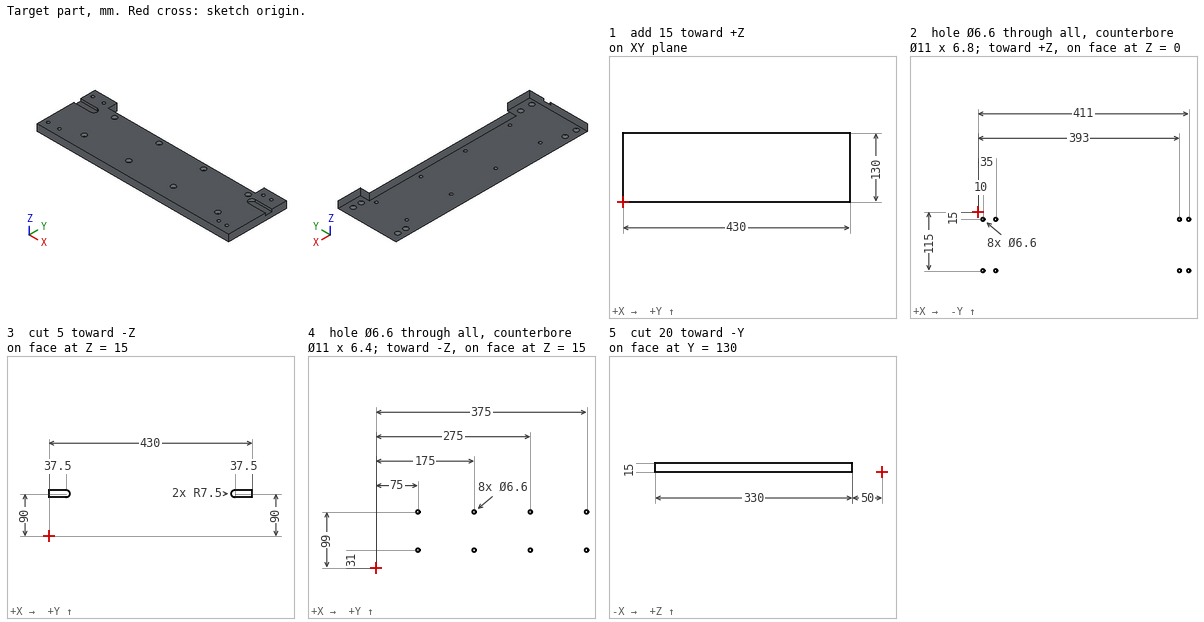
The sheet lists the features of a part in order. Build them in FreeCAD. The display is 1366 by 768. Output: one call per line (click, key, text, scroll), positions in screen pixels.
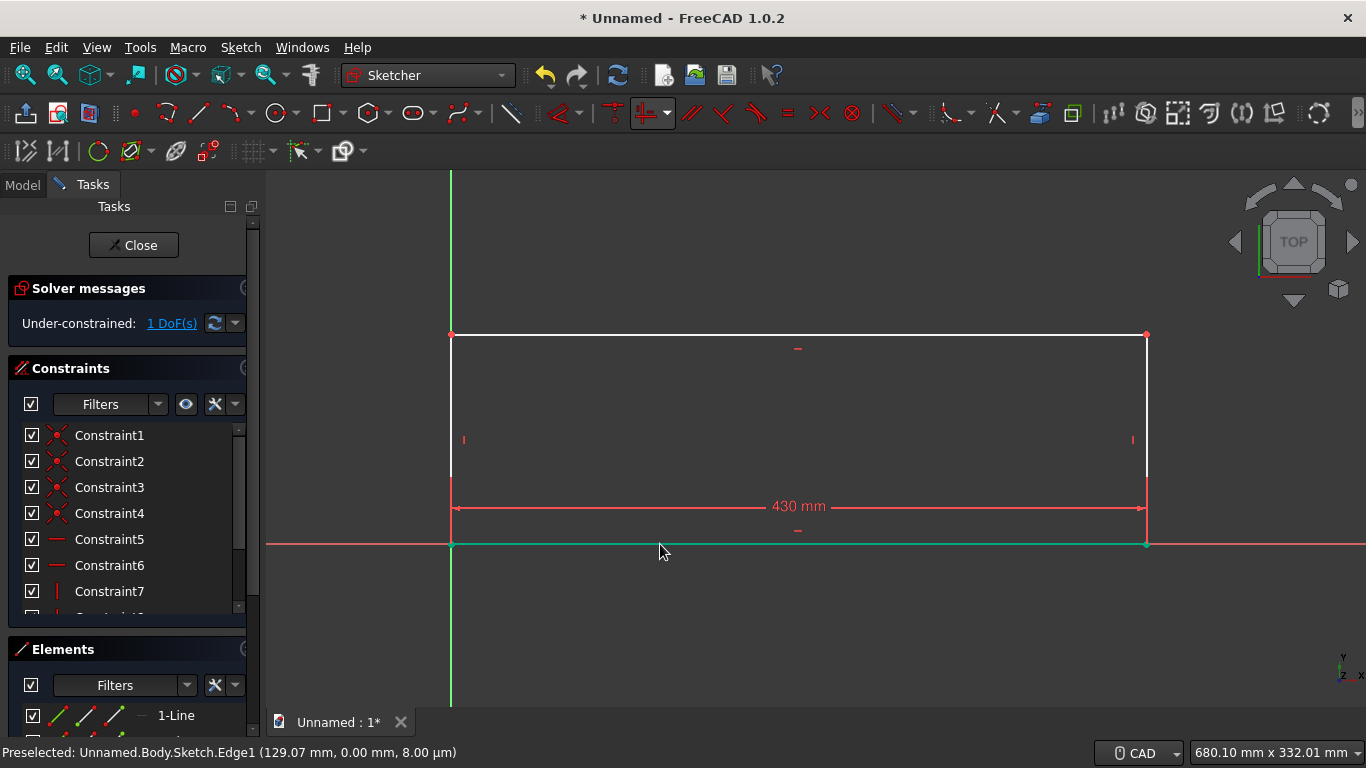
click(1147, 481)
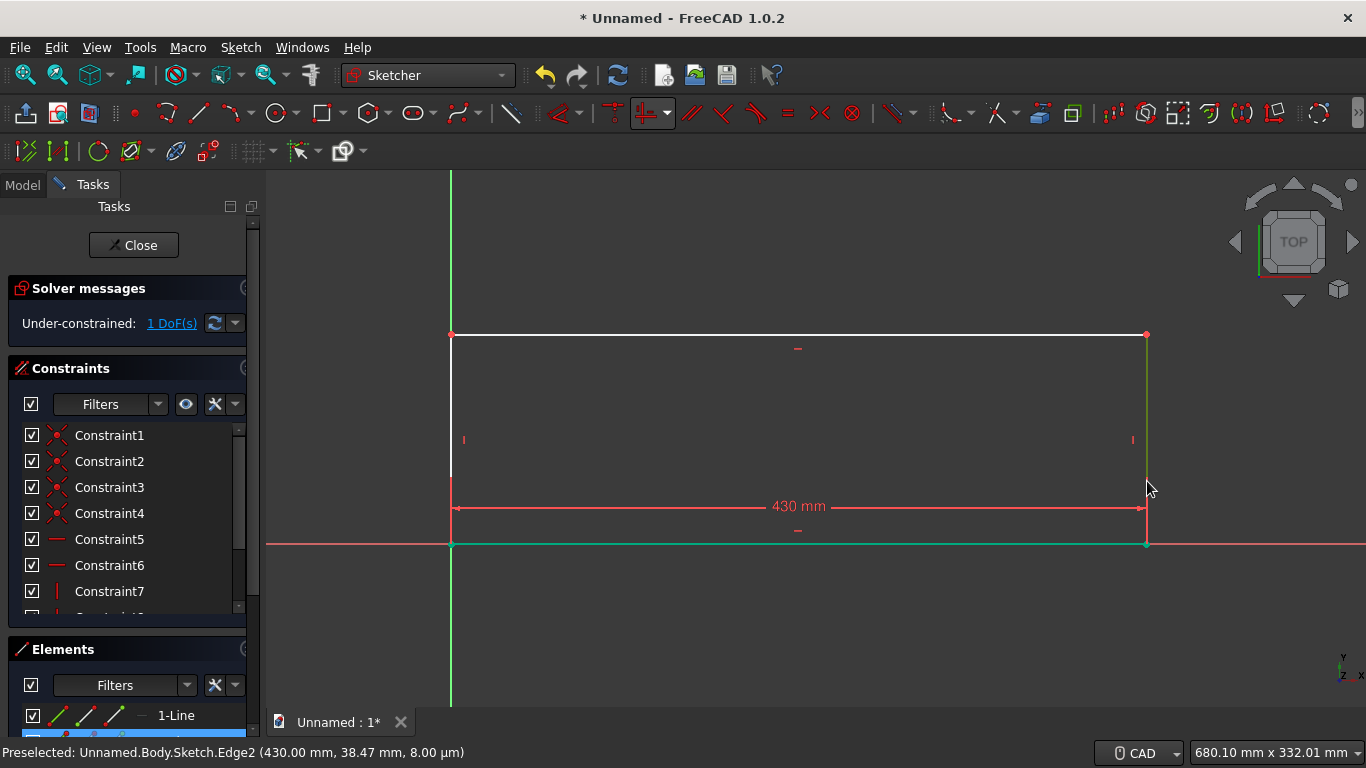
key(i)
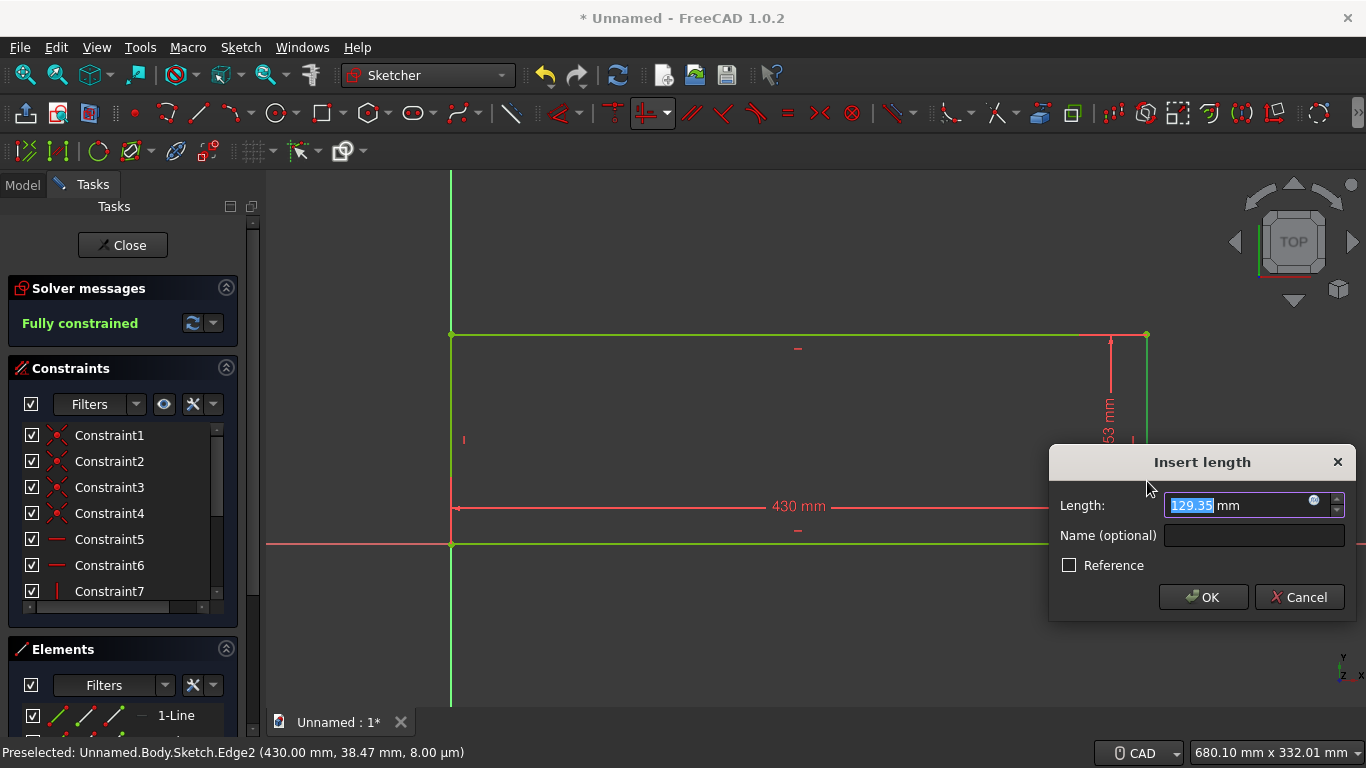
text(130)
key(Return)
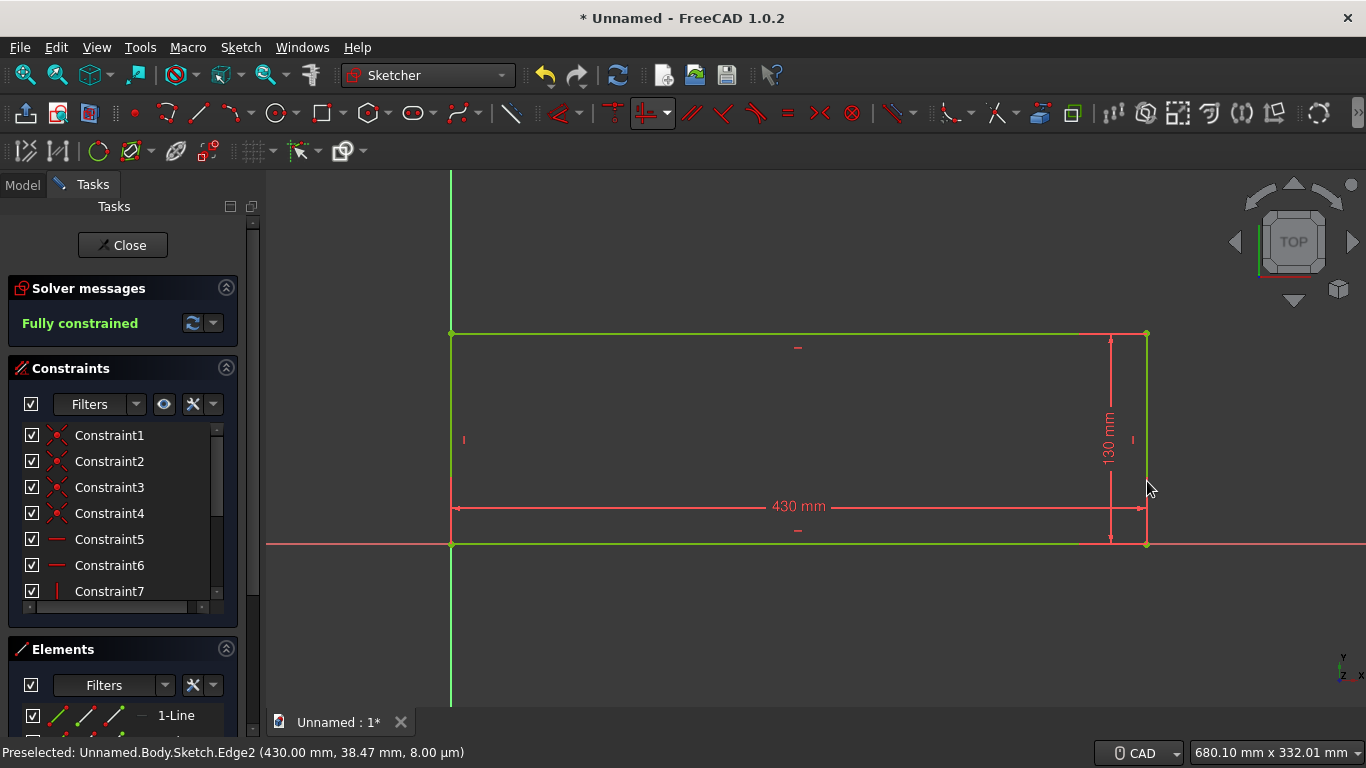
click(123, 245)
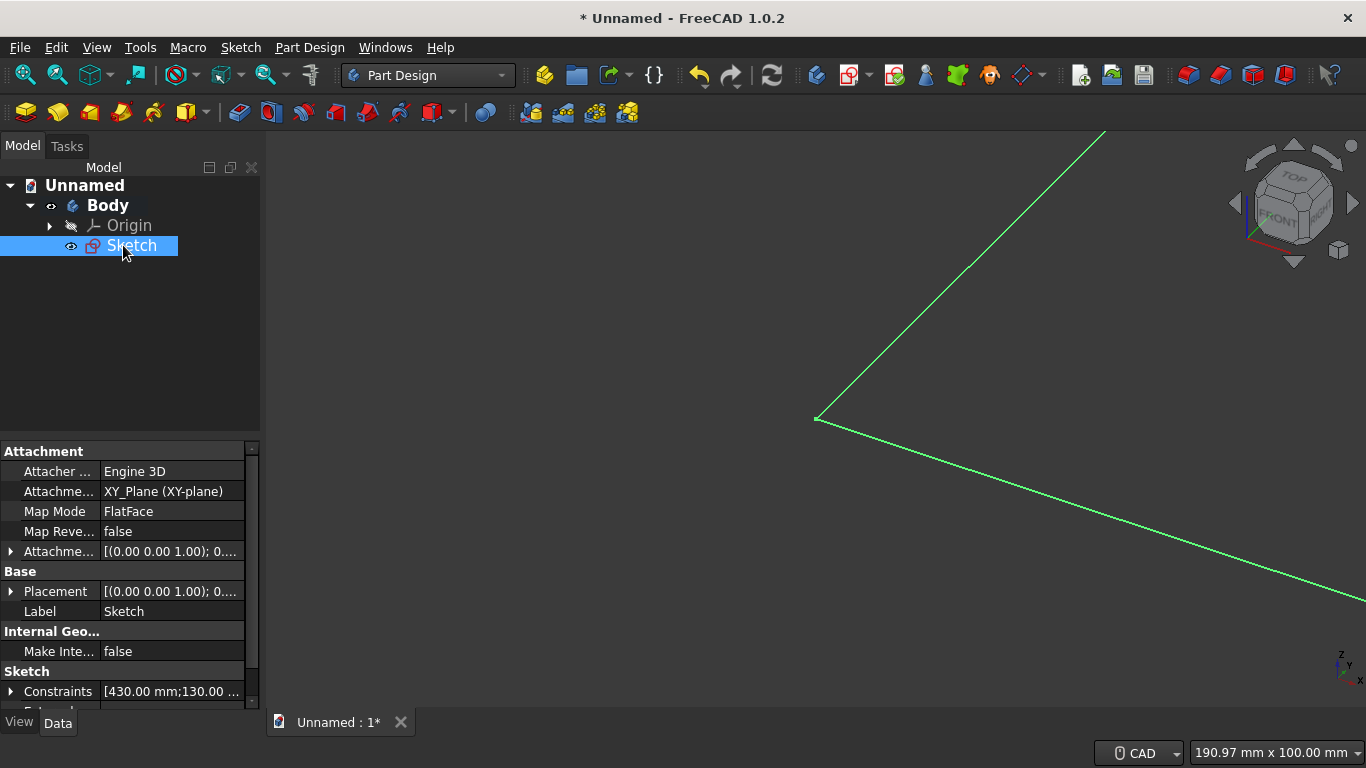
click(26, 112)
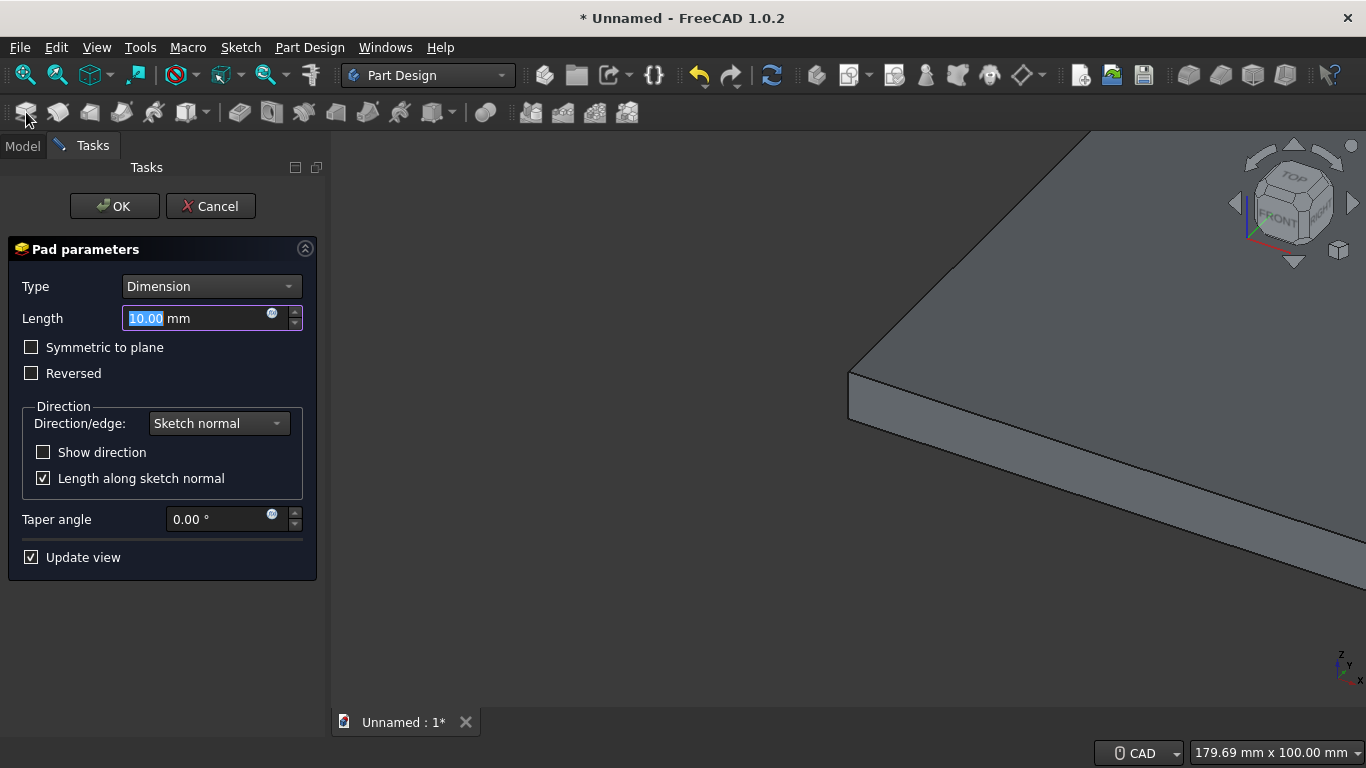
text(15)
key(Tab)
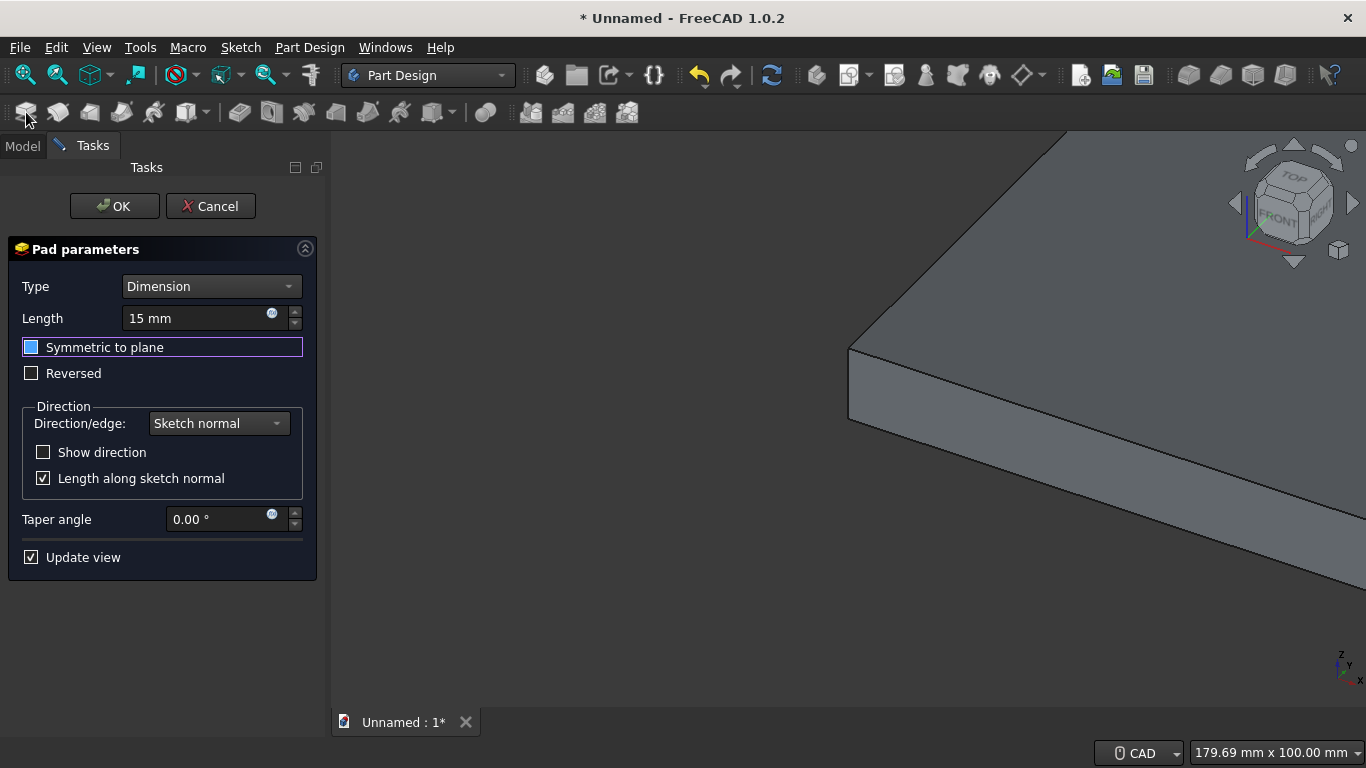
click(115, 206)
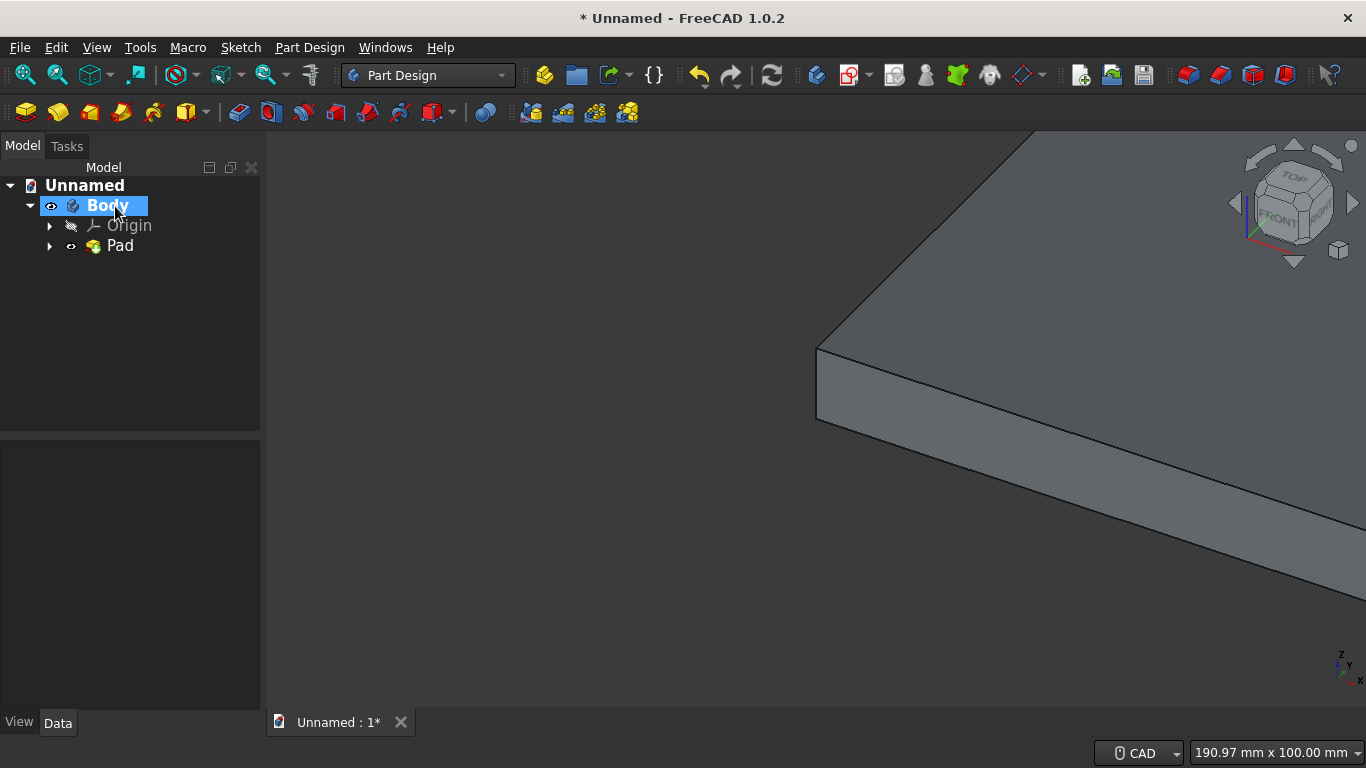
click(26, 76)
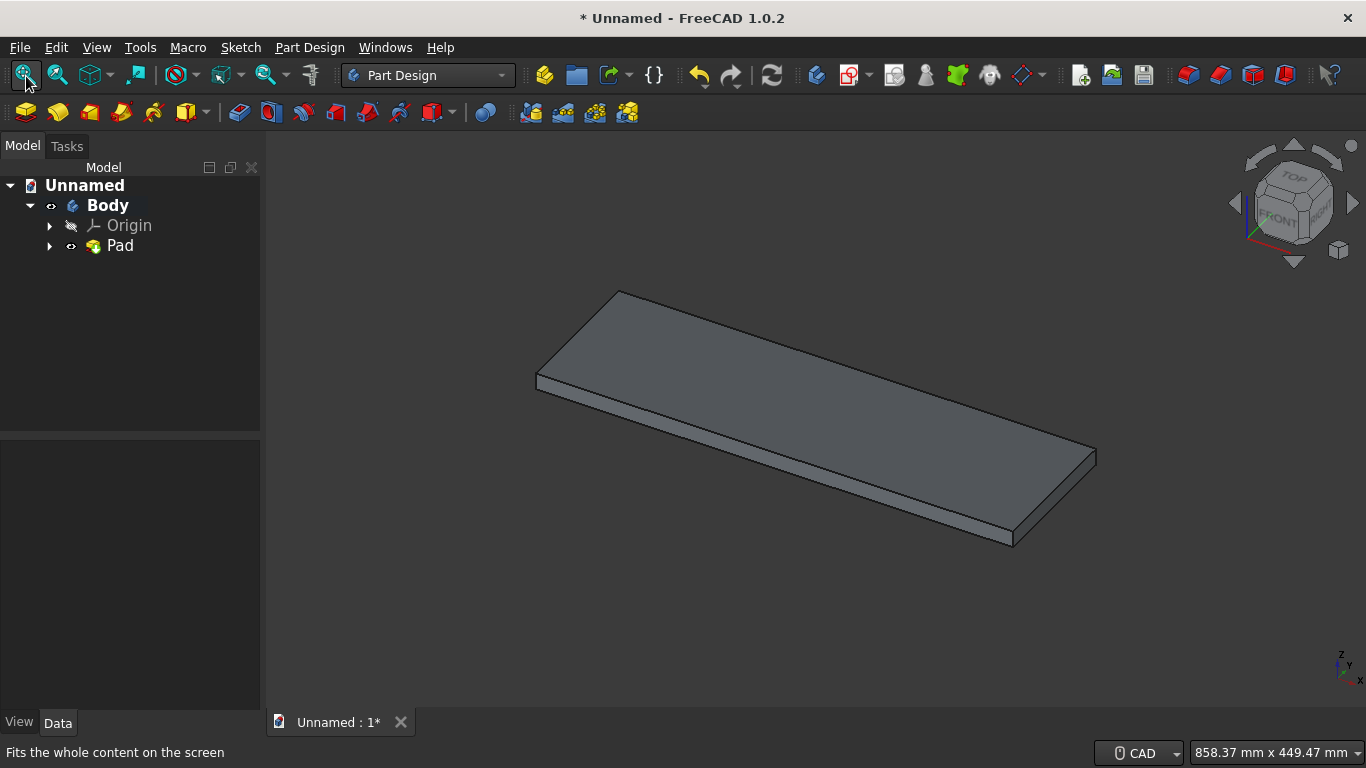
key(5)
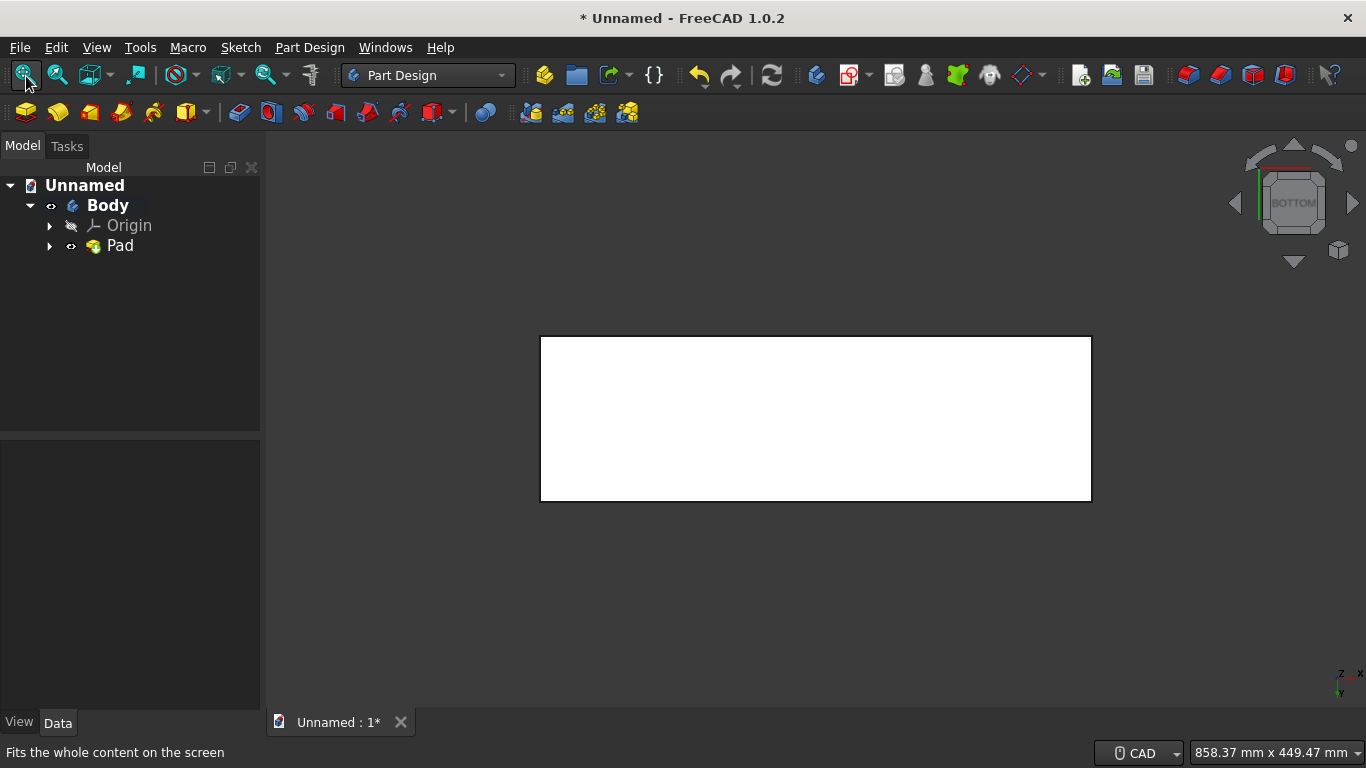
click(973, 418)